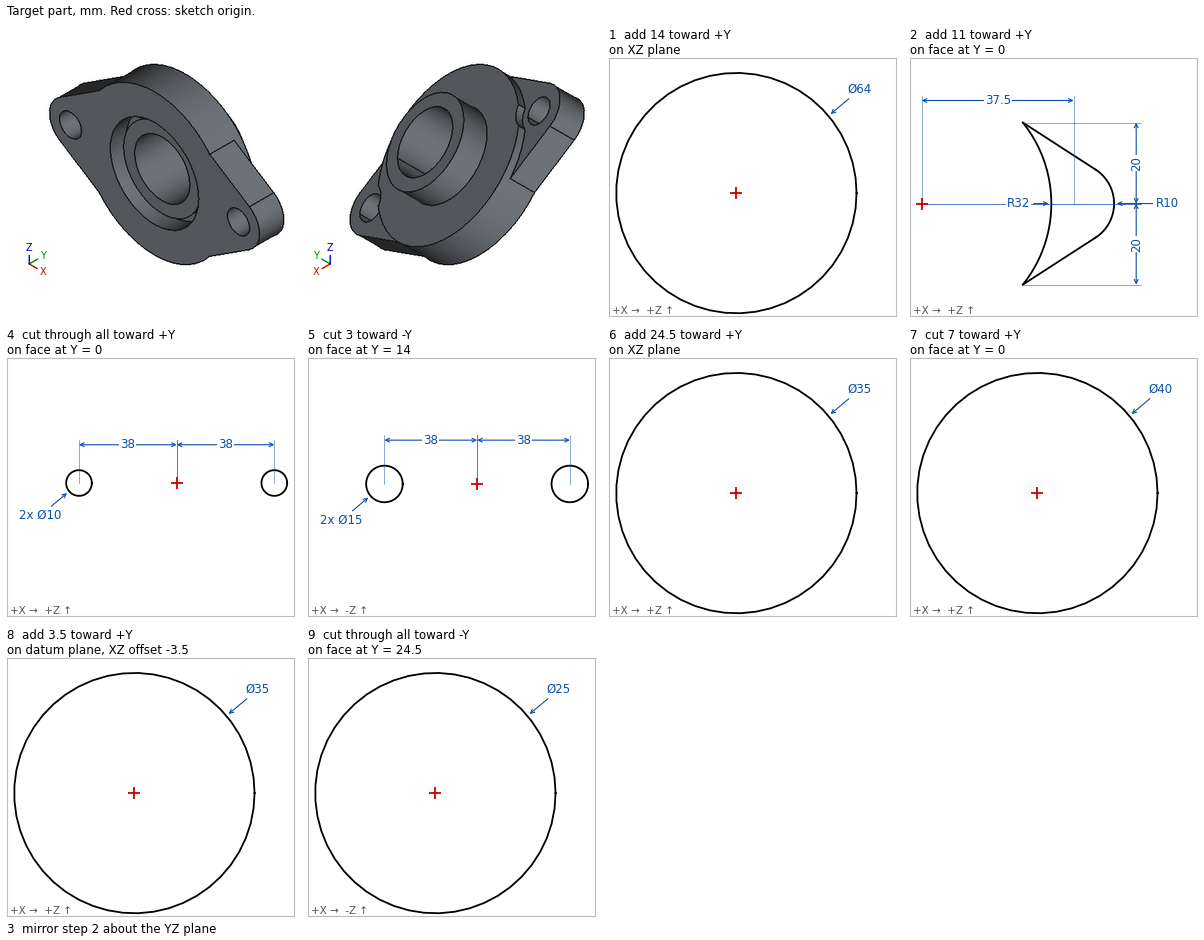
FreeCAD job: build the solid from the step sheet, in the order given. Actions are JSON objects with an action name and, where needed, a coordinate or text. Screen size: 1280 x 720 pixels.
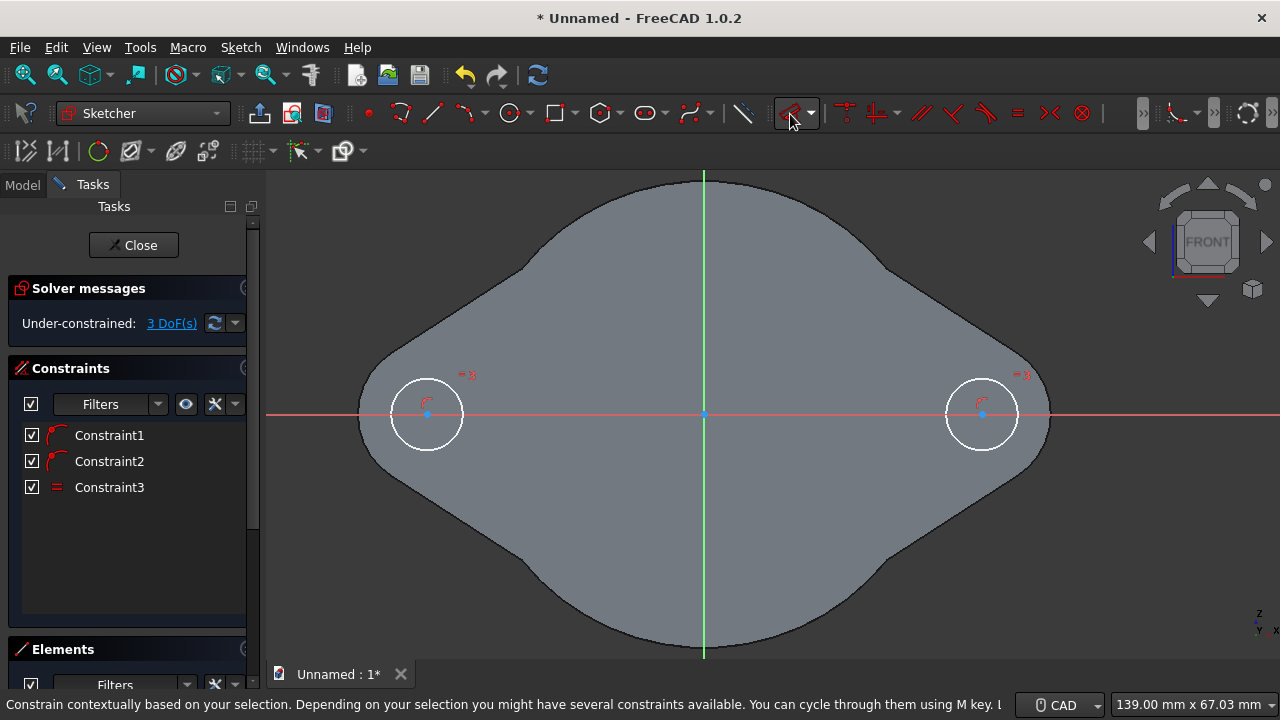
{"action": "left_click", "coordinate": [452, 389]}
{"action": "left_click", "coordinate": [474, 366]}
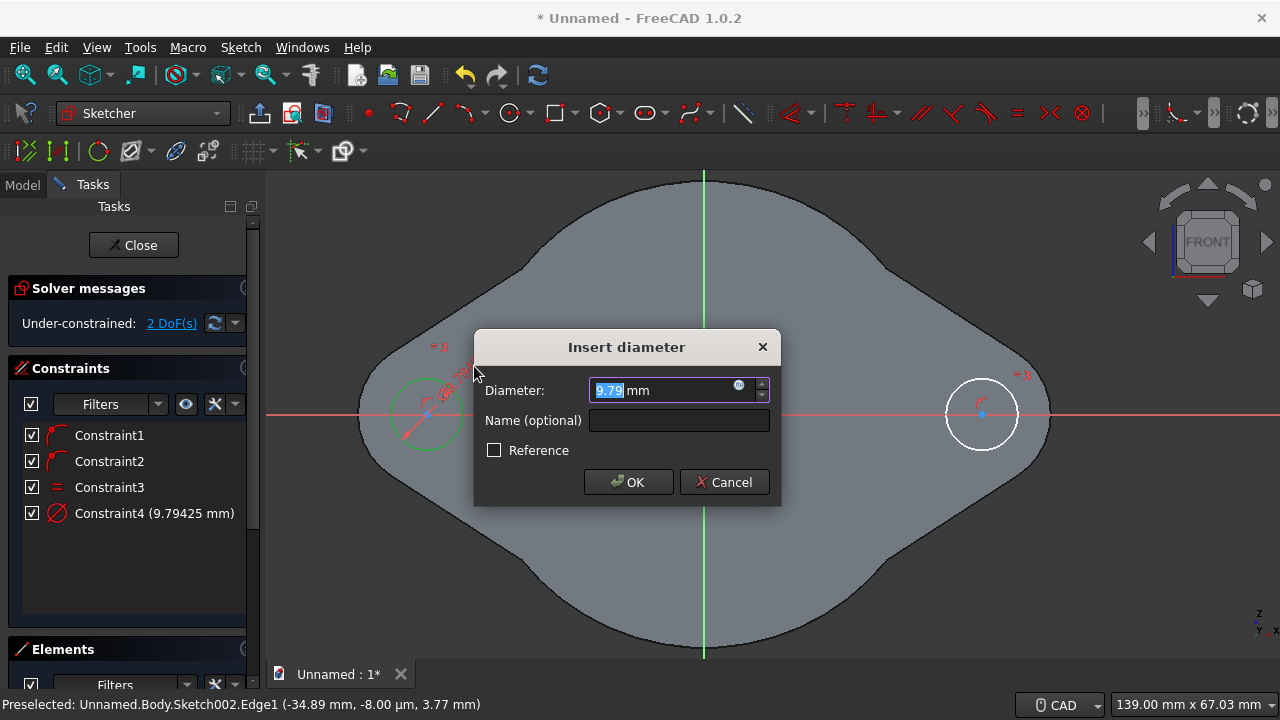
{"action": "type", "text": "10"}
{"action": "key", "text": "Return"}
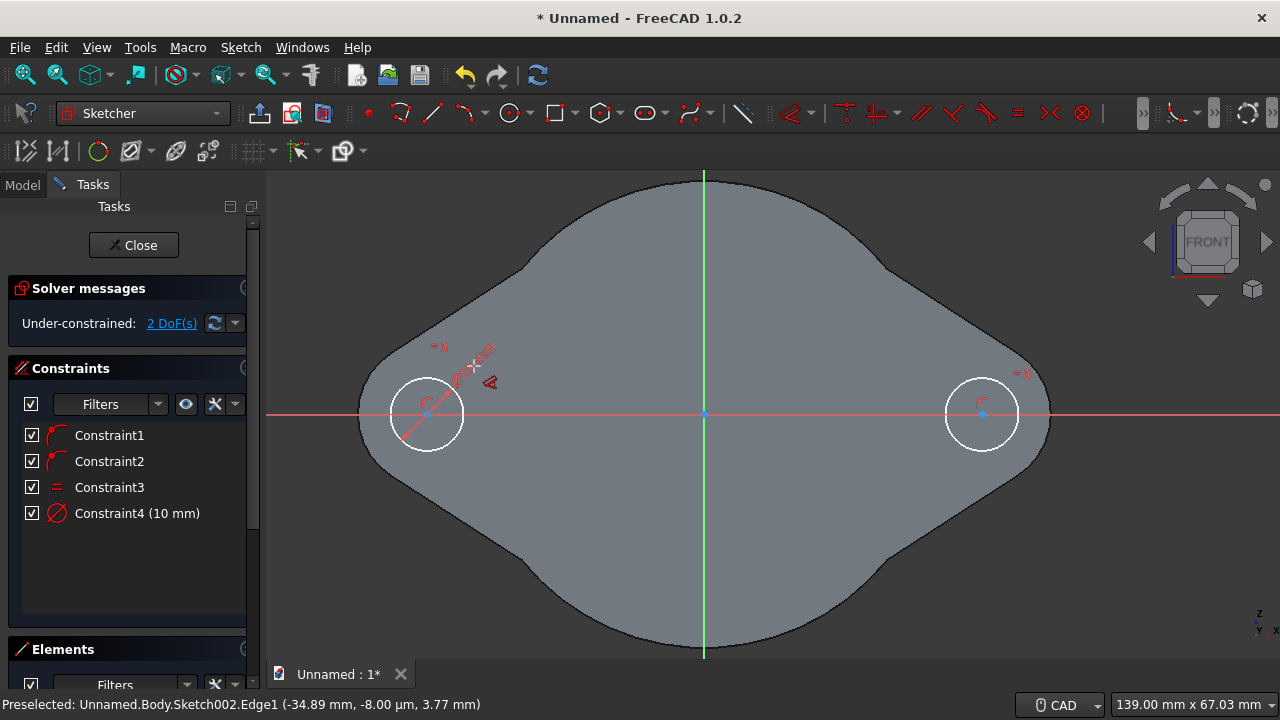
{"action": "left_click", "coordinate": [427, 414]}
{"action": "left_click", "coordinate": [566, 448]}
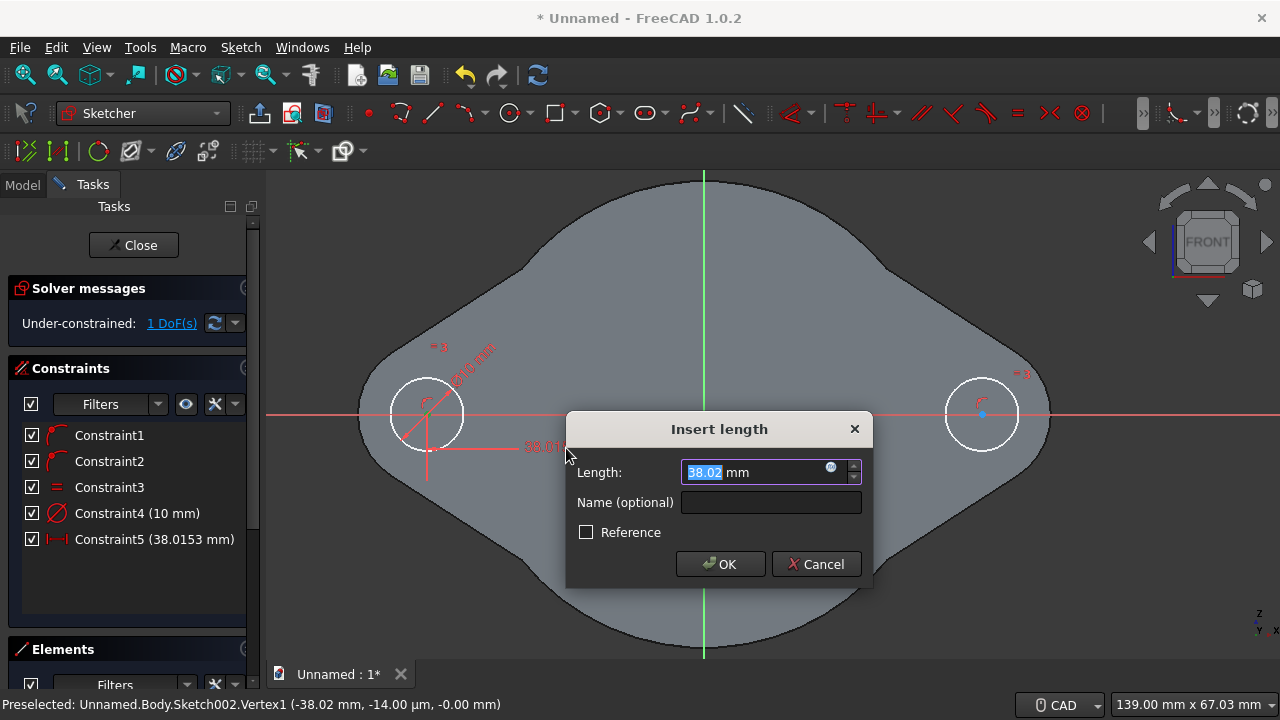
{"action": "type", "text": "38"}
{"action": "key", "text": "Return"}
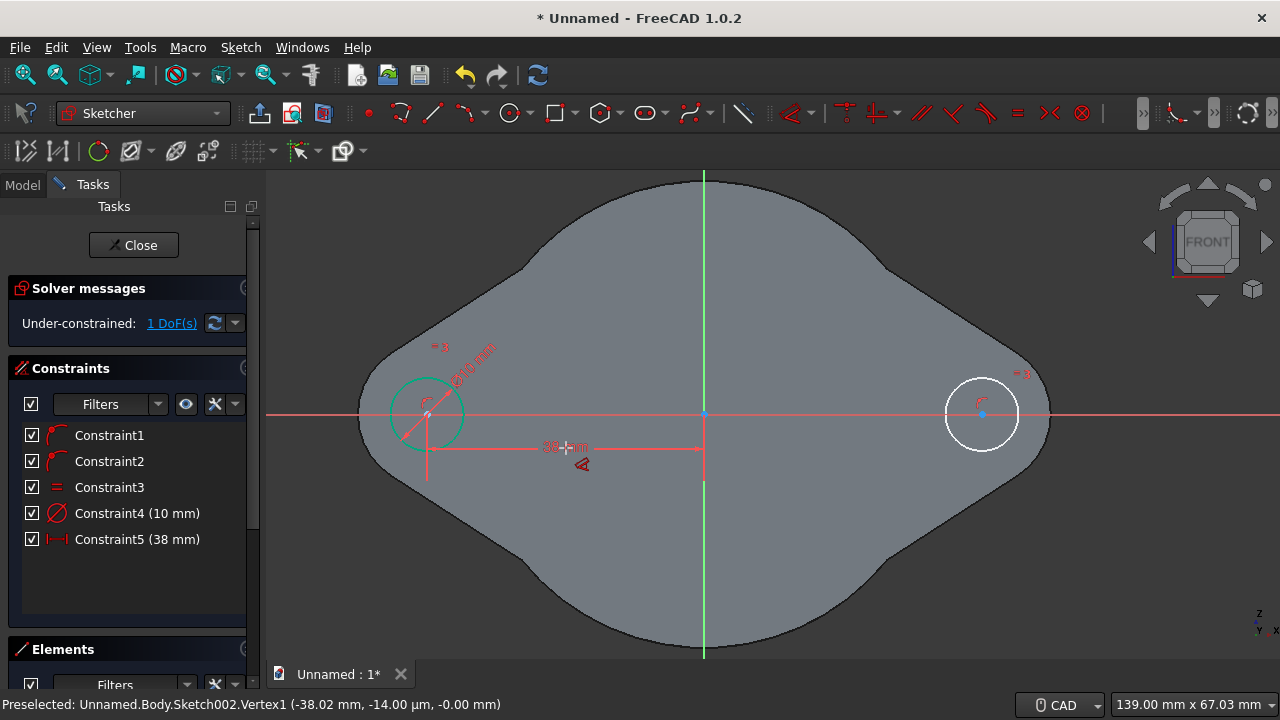
{"action": "left_click", "coordinate": [982, 414]}
{"action": "left_click", "coordinate": [843, 448]}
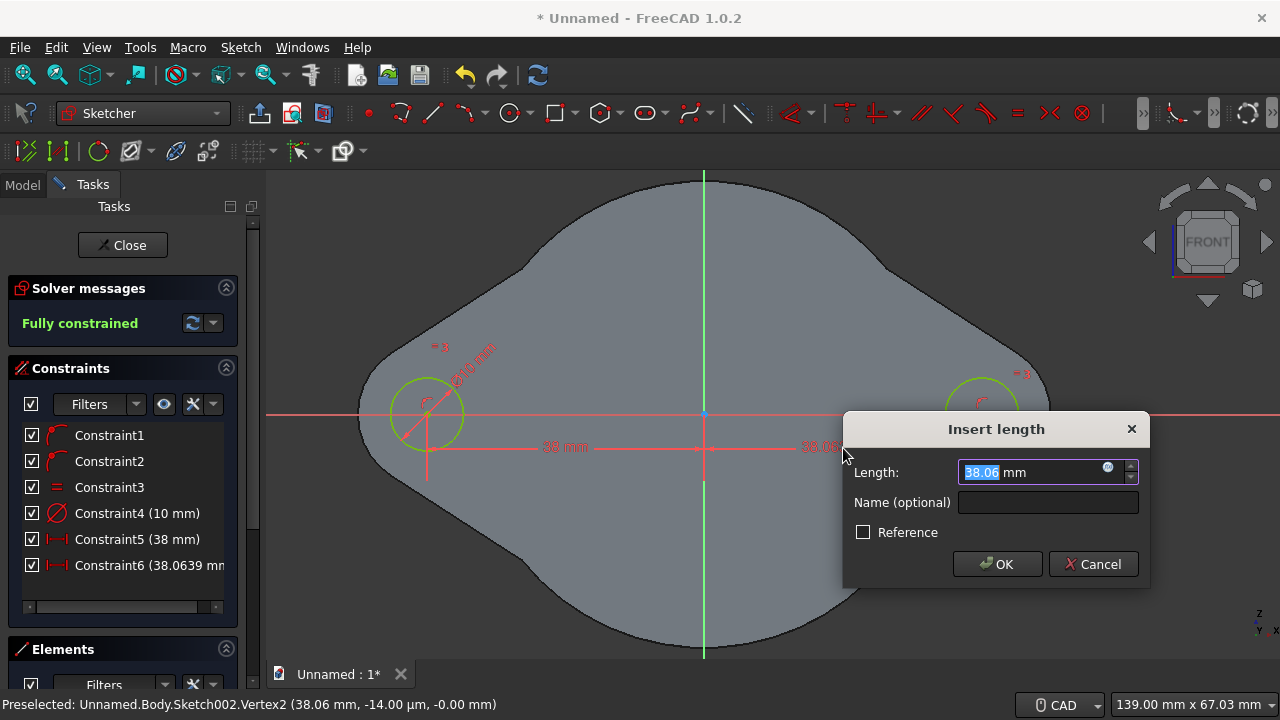
{"action": "type", "text": "38"}
{"action": "key", "text": "Return"}
{"action": "key", "text": "Escape"}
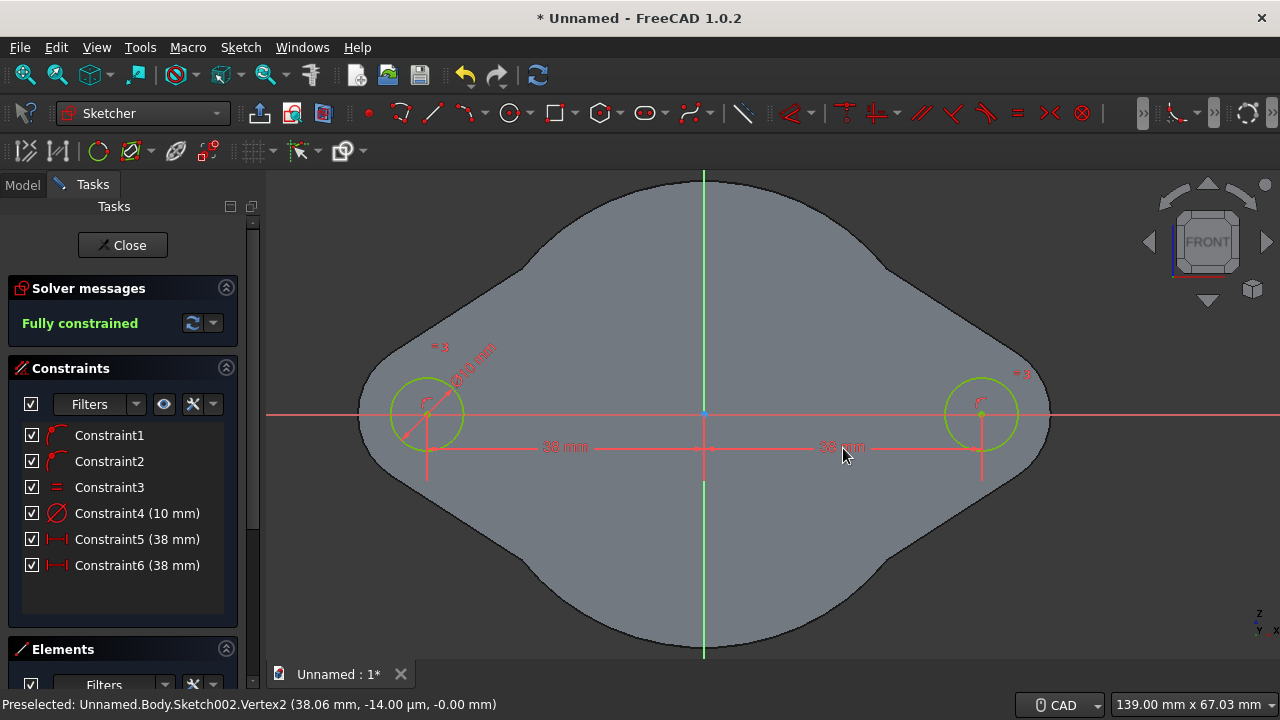
{"action": "left_click", "coordinate": [123, 245]}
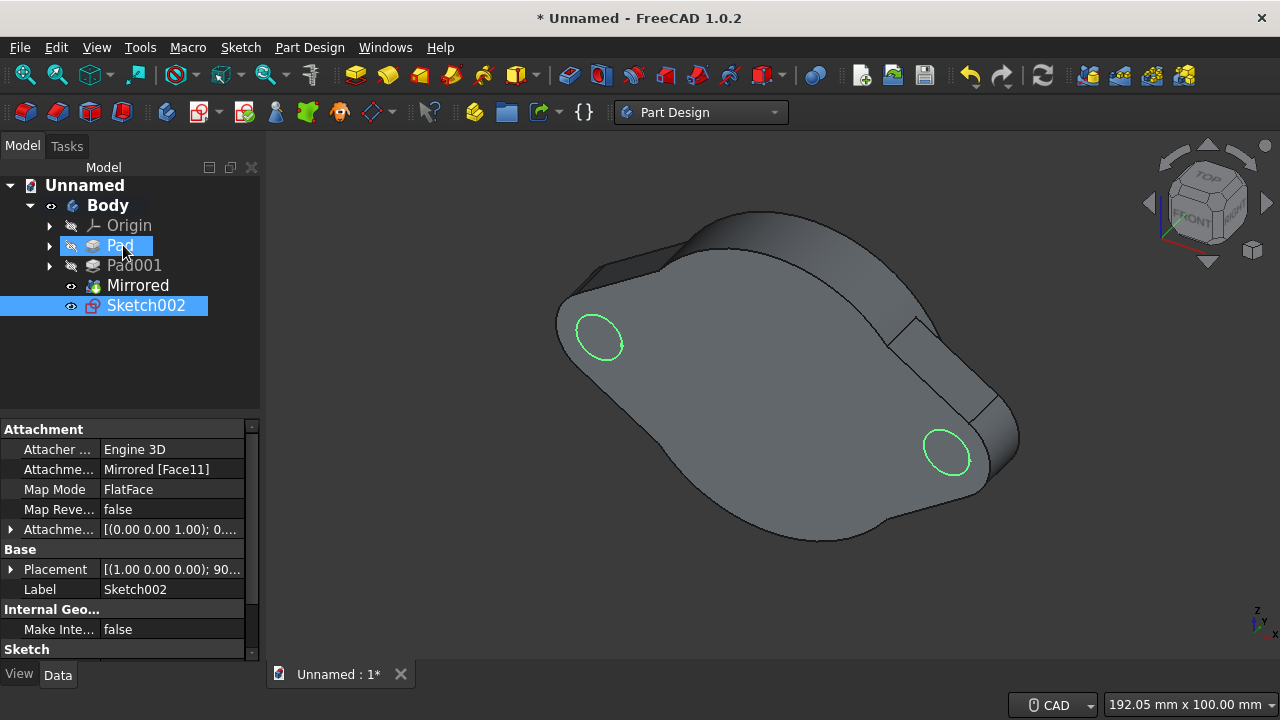
{"action": "left_click", "coordinate": [570, 76]}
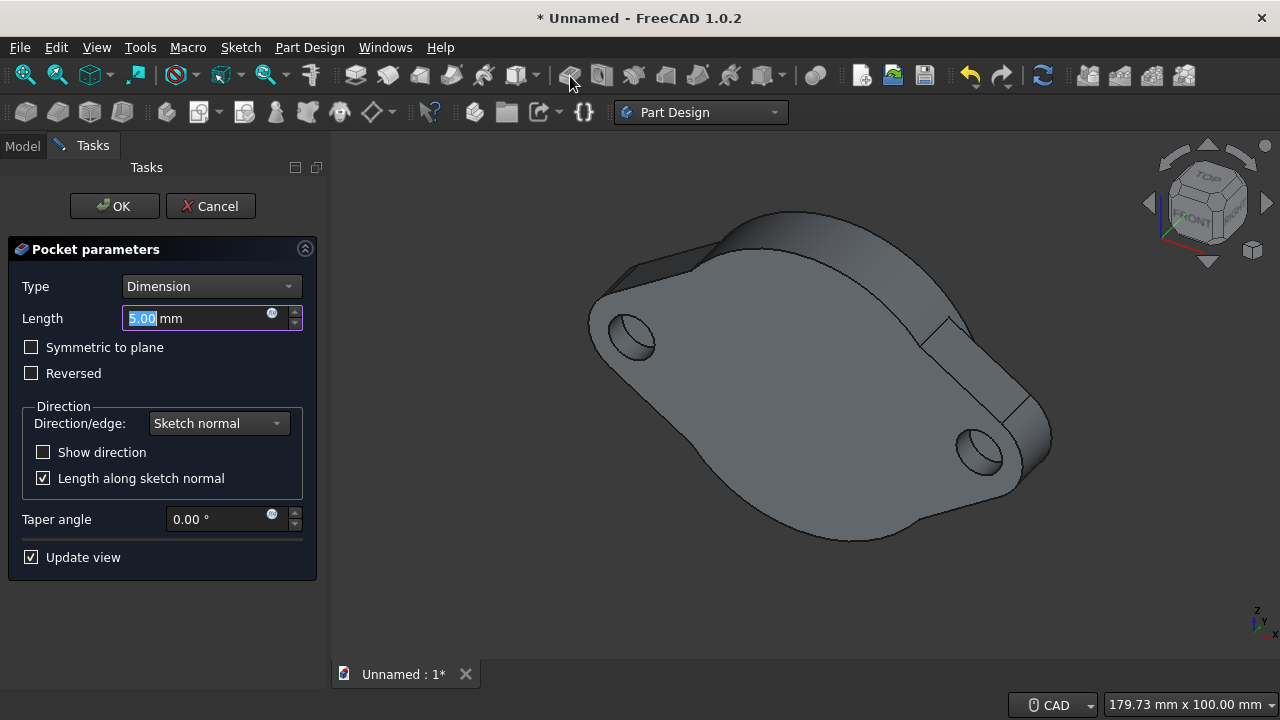
{"action": "left_click", "coordinate": [212, 286]}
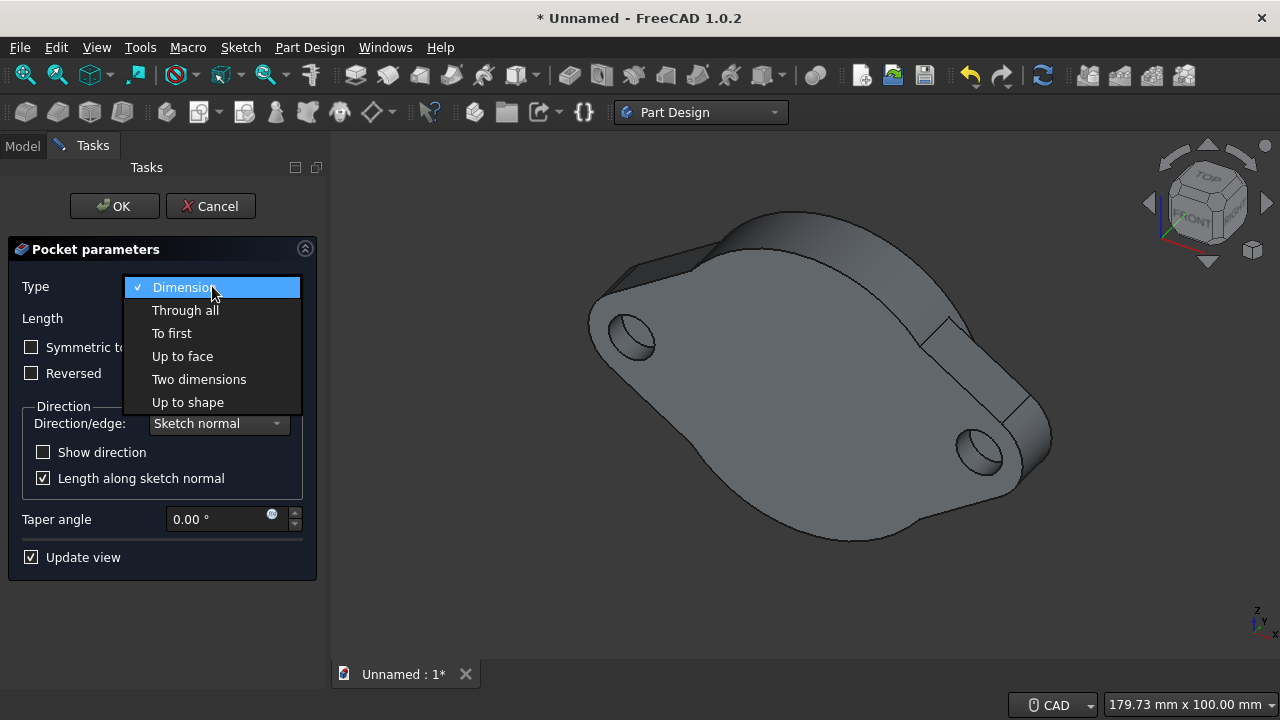
{"action": "left_click", "coordinate": [212, 310]}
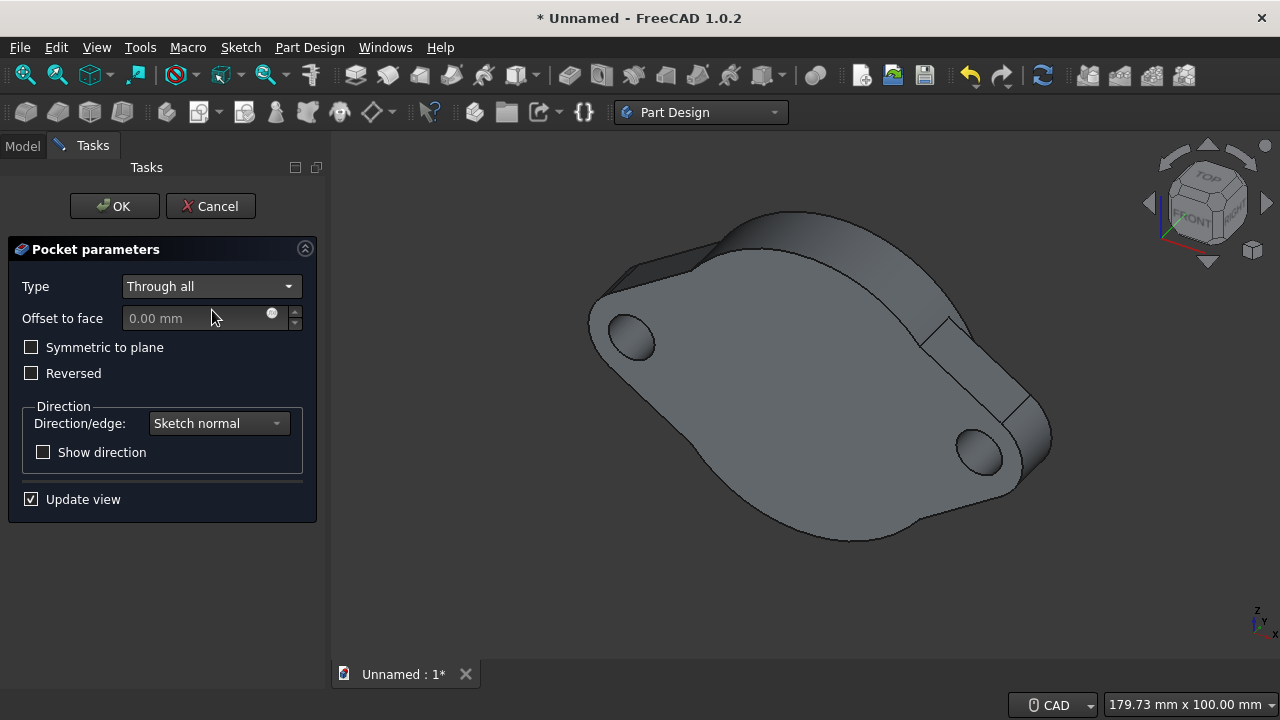
{"action": "left_click", "coordinate": [115, 206]}